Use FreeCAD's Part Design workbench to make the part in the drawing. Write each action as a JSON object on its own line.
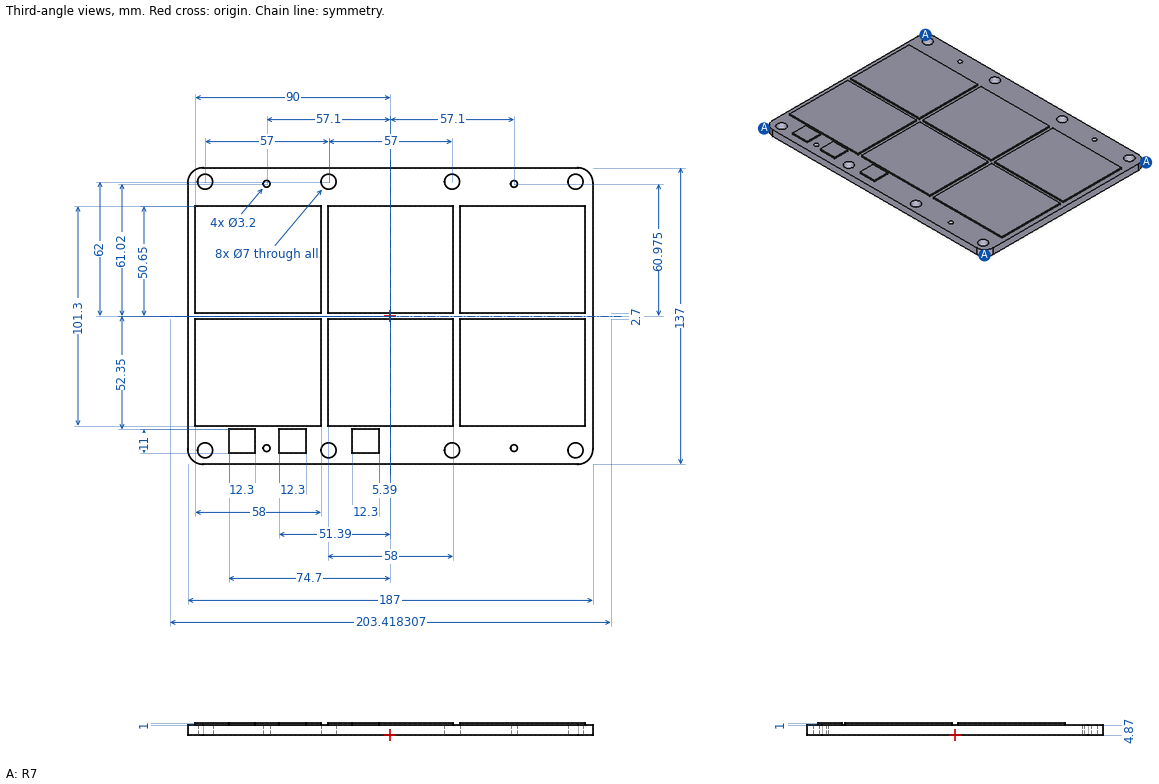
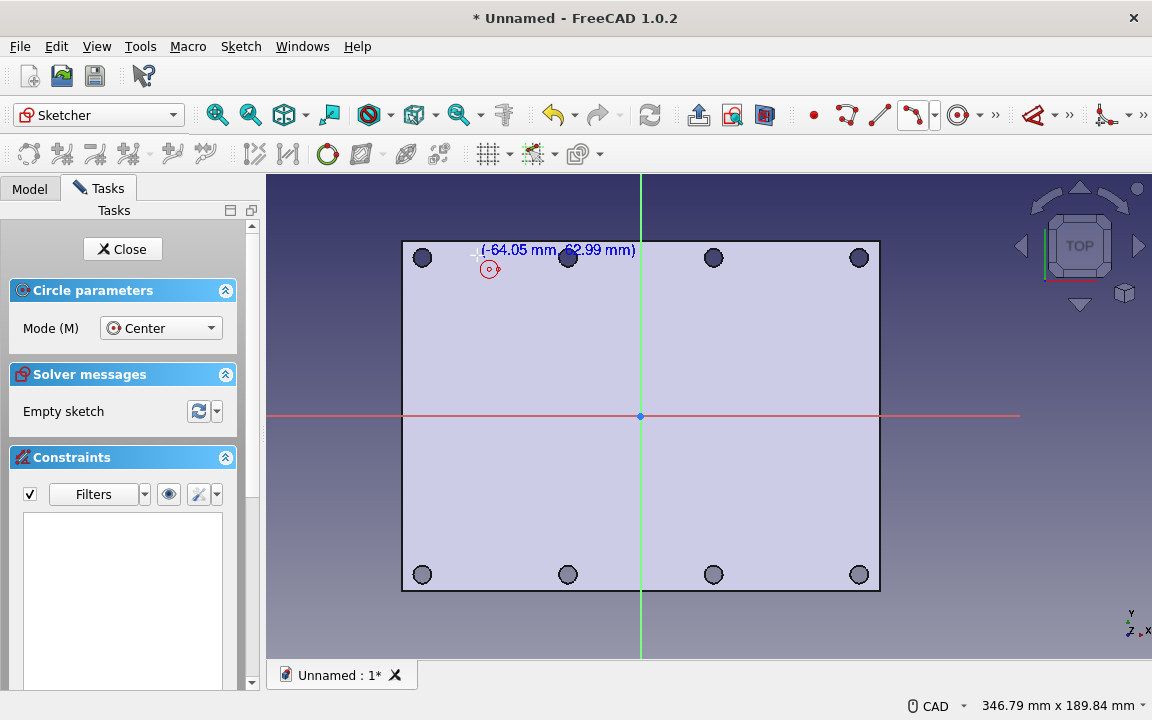
{"action": "left_click", "coordinate": [495, 260]}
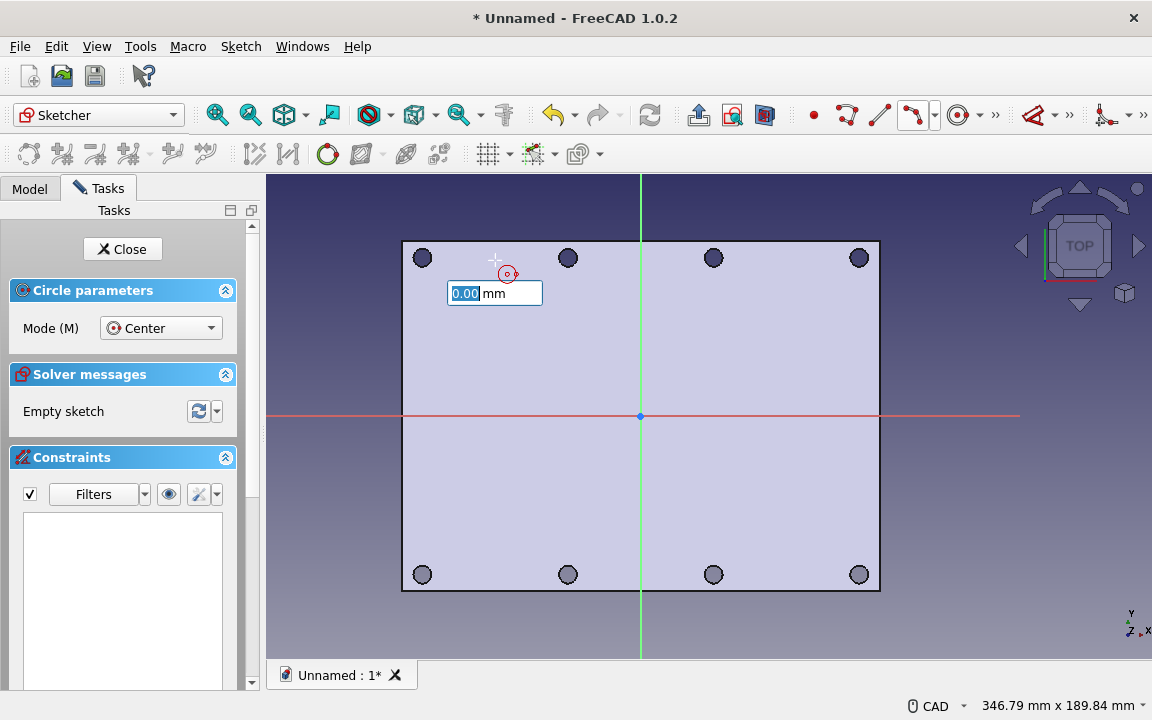
{"action": "scroll", "coordinate": [498, 257], "scroll_direction": "up", "scroll_amount": 7}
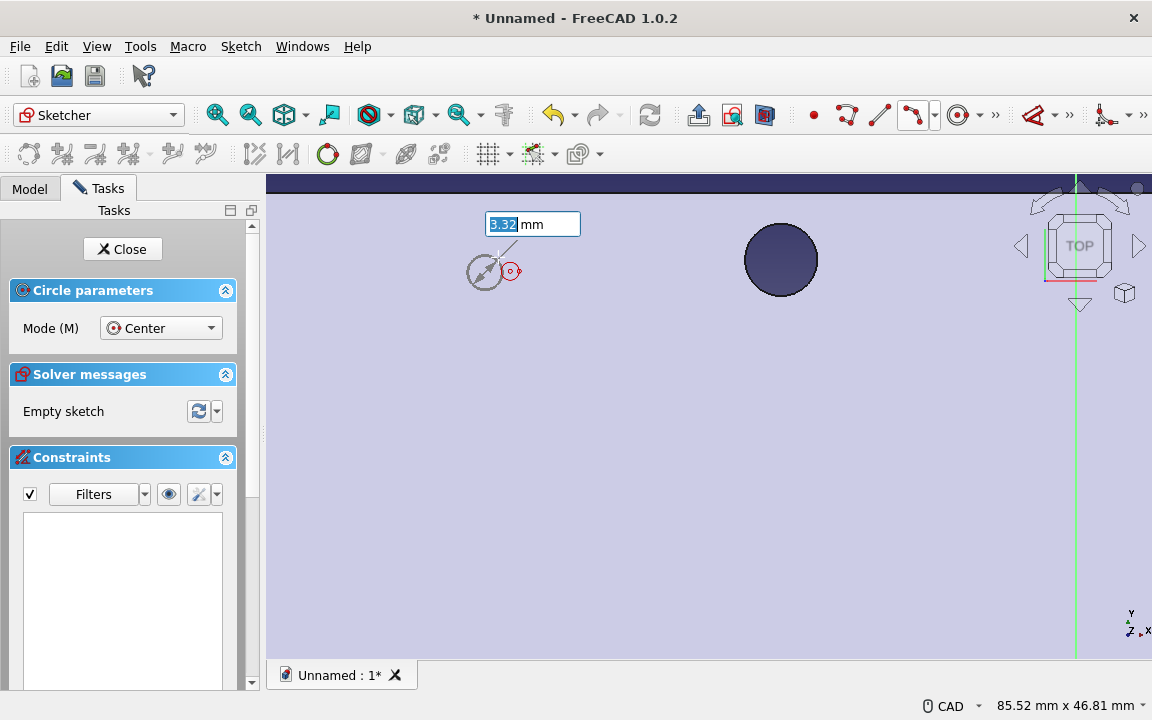
{"action": "left_click", "coordinate": [497, 258]}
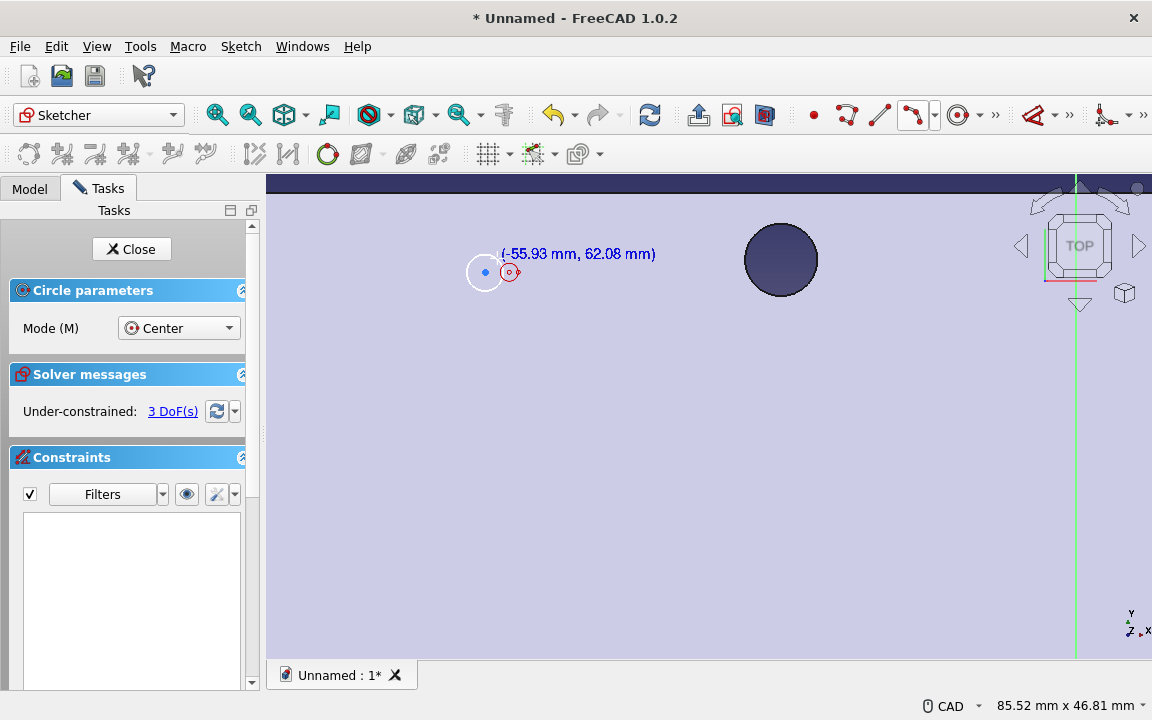
{"action": "scroll", "coordinate": [498, 258], "scroll_direction": "down", "scroll_amount": 7}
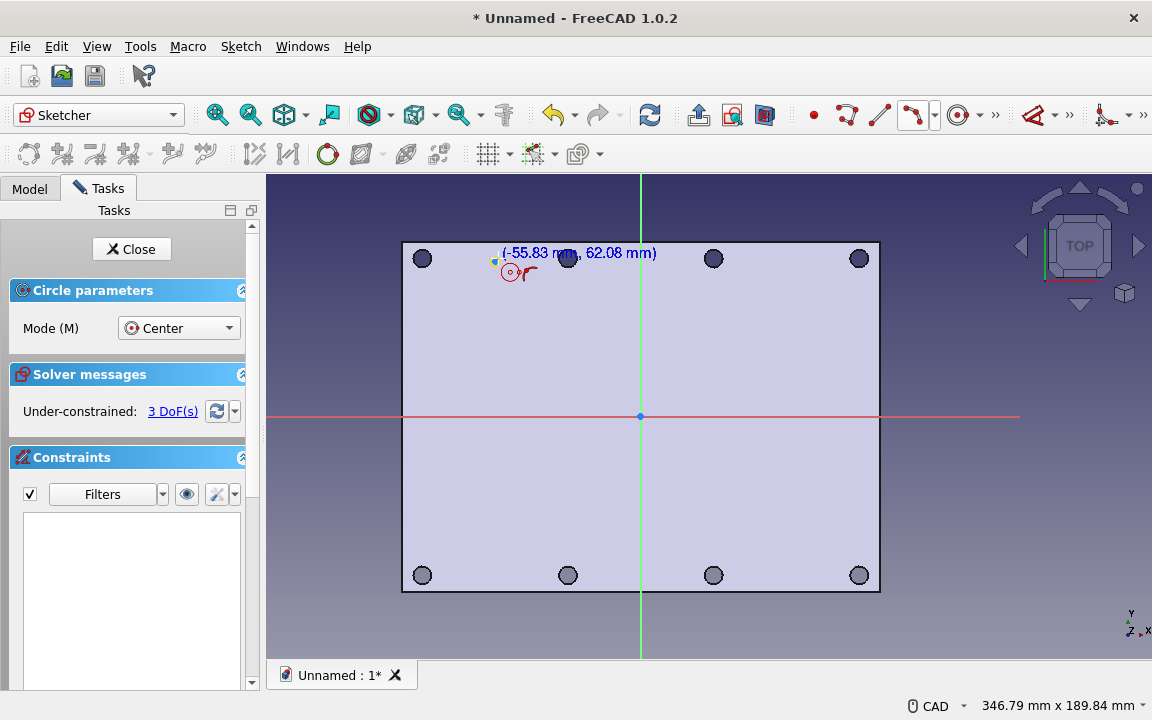
{"action": "scroll", "coordinate": [787, 261], "scroll_direction": "up", "scroll_amount": 9}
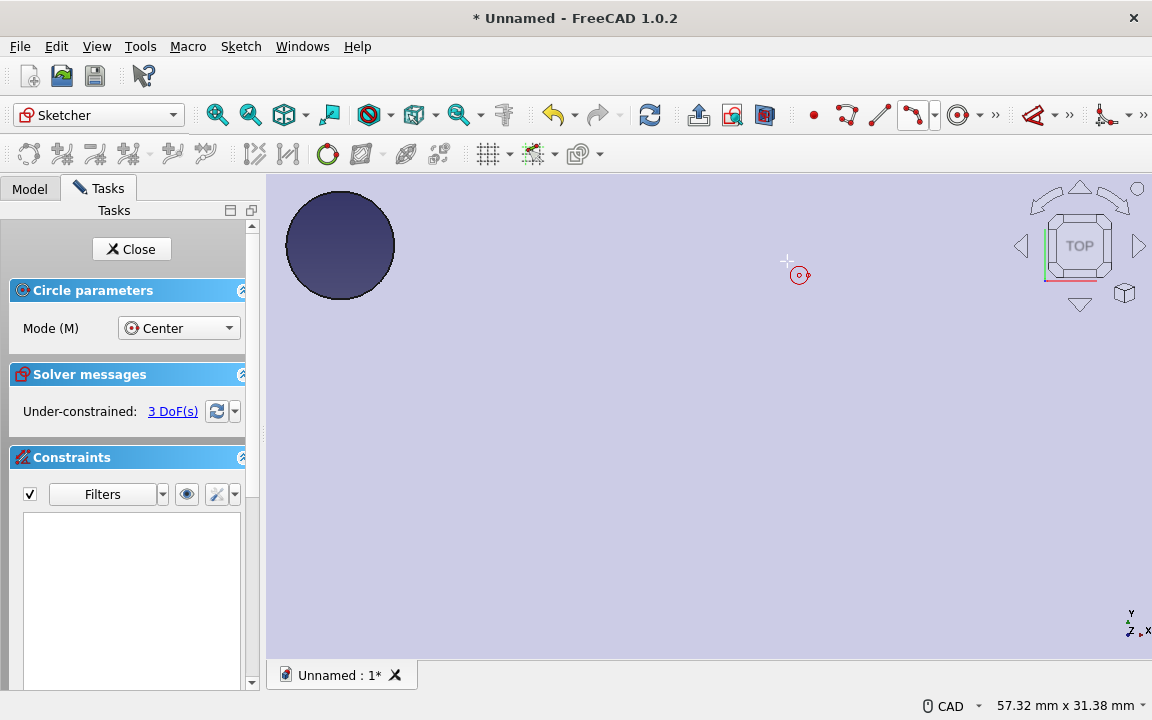
{"action": "scroll", "coordinate": [787, 261], "scroll_direction": "down", "scroll_amount": 9}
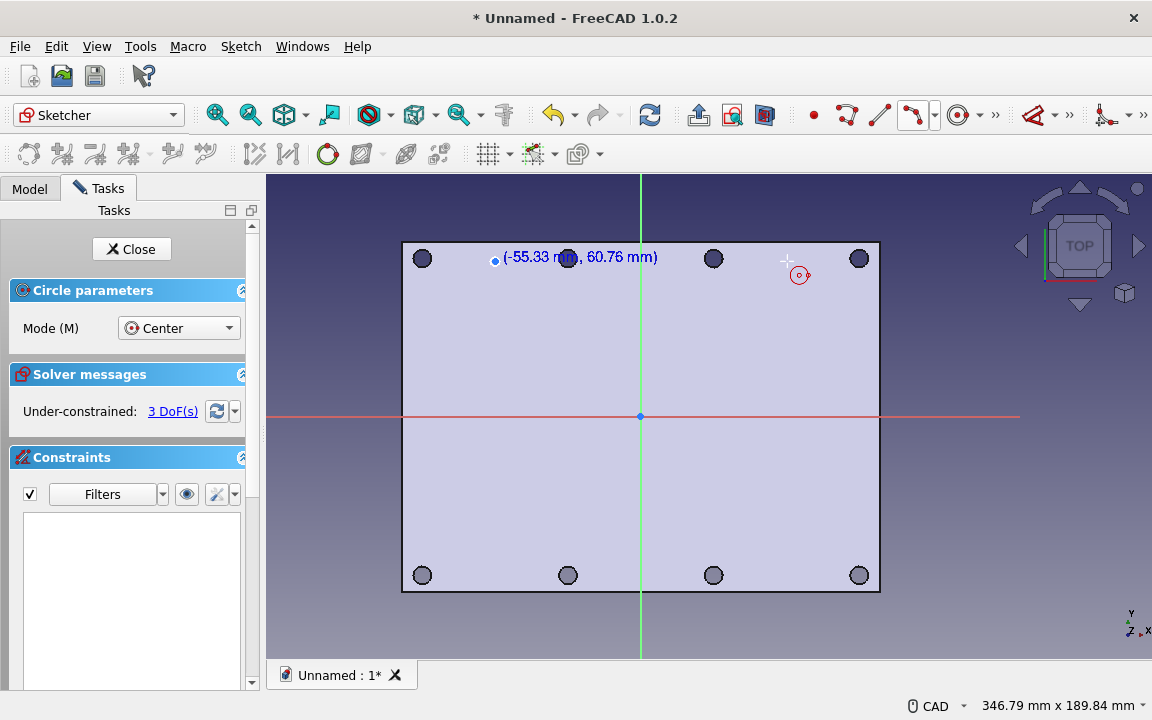
{"action": "left_click", "coordinate": [787, 261]}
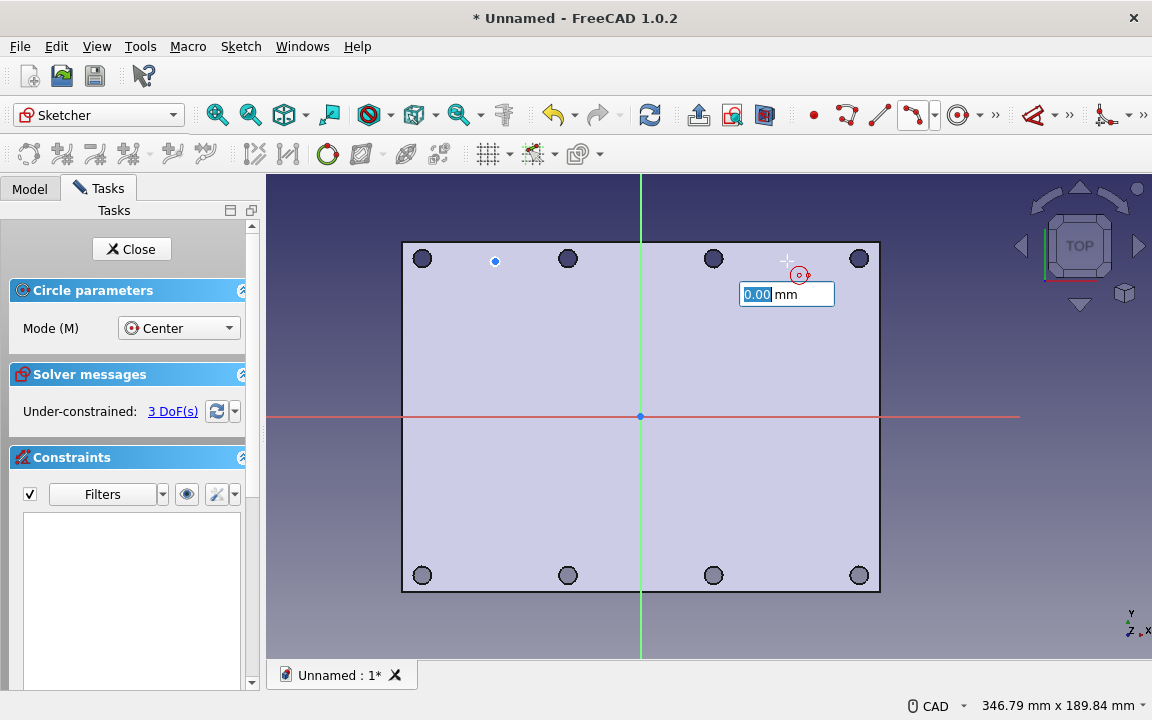
{"action": "scroll", "coordinate": [790, 258], "scroll_direction": "up", "scroll_amount": 7}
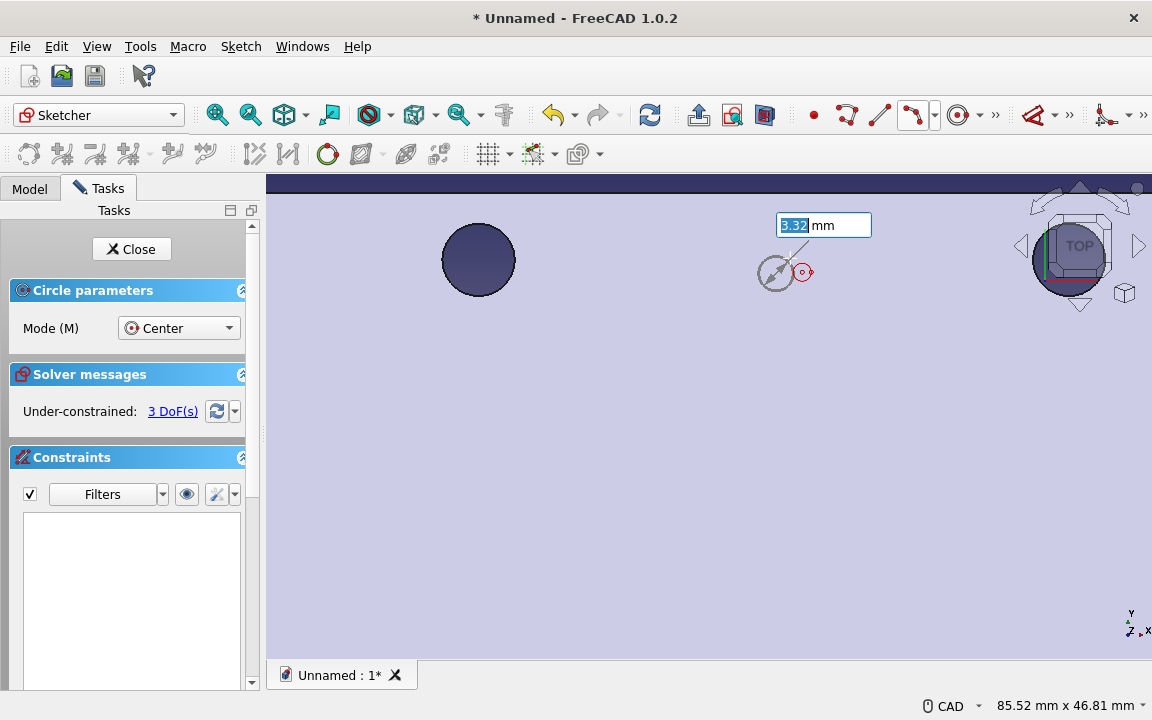
{"action": "left_click", "coordinate": [787, 259]}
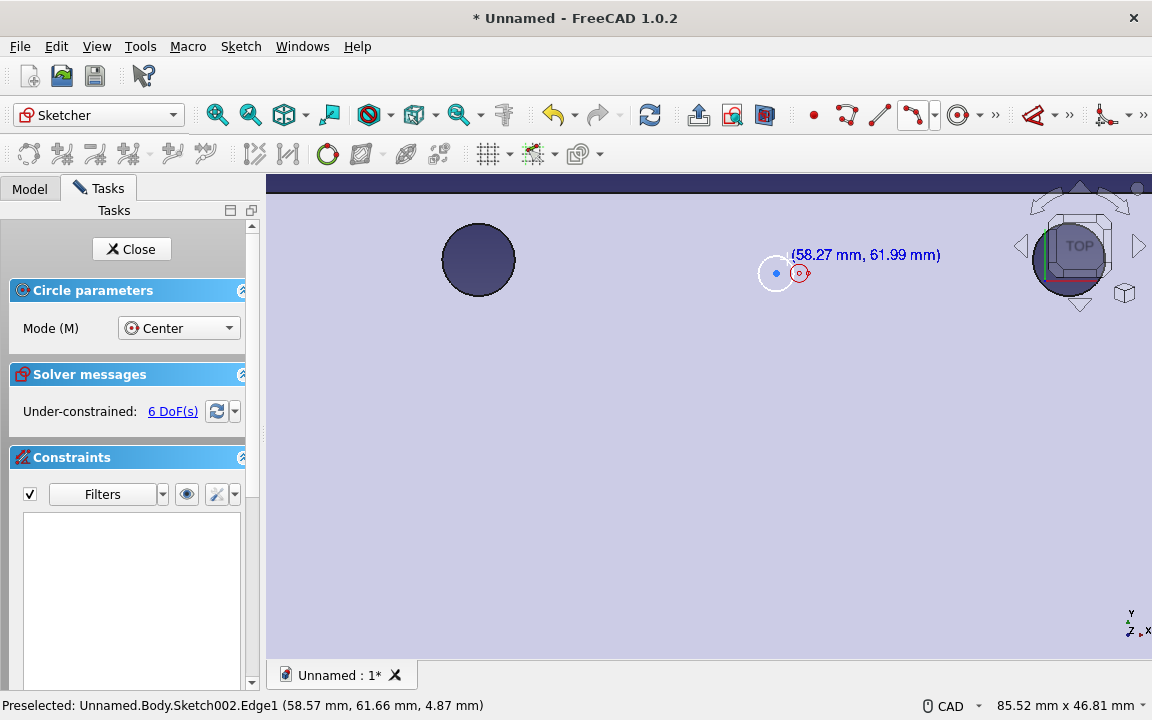
{"action": "scroll", "coordinate": [790, 258], "scroll_direction": "down", "scroll_amount": 7}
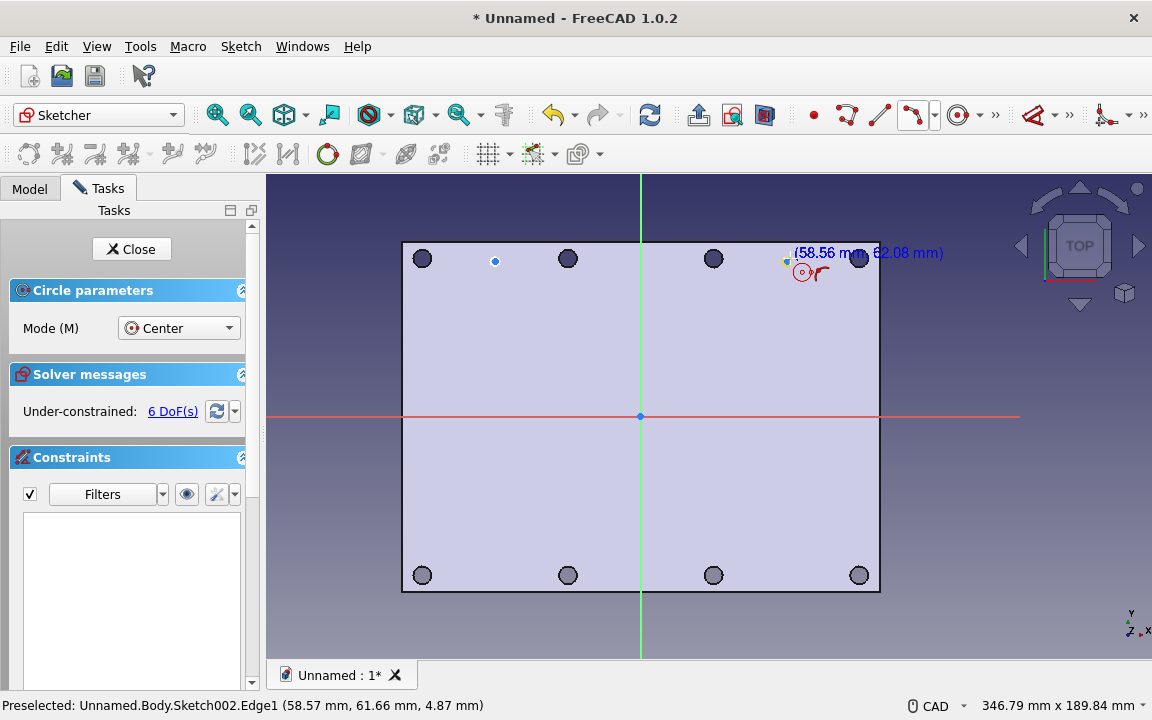
{"action": "scroll", "coordinate": [787, 573], "scroll_direction": "up", "scroll_amount": 9}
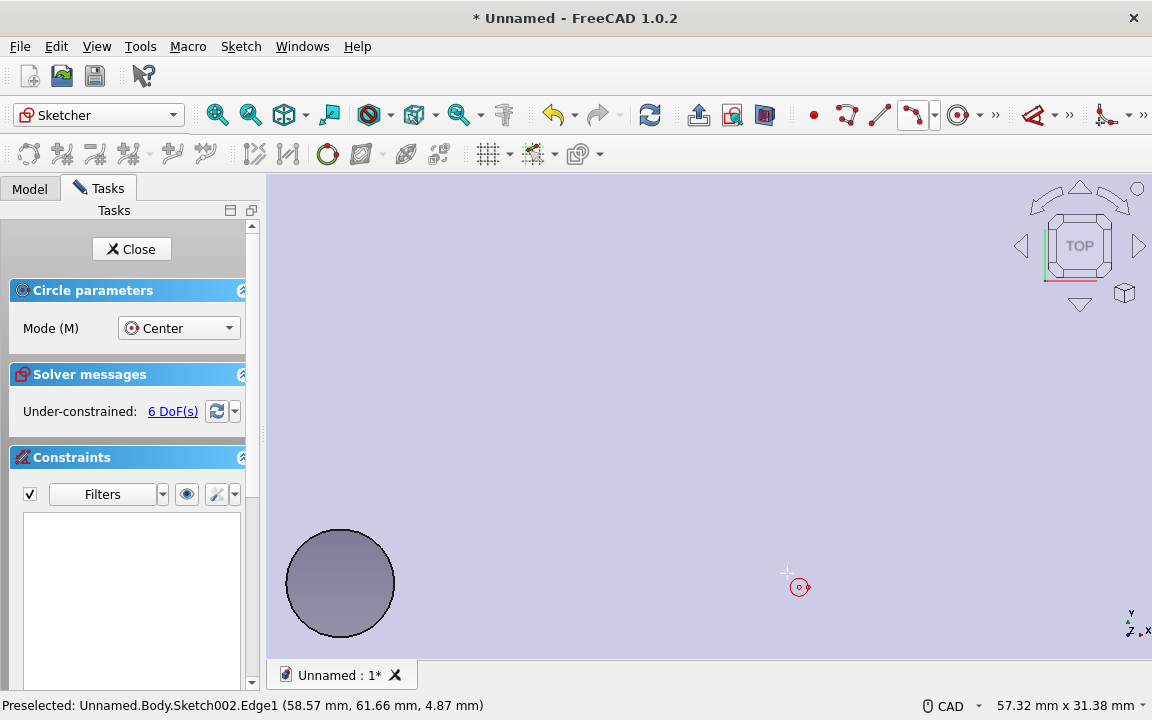
{"action": "scroll", "coordinate": [787, 573], "scroll_direction": "down", "scroll_amount": 9}